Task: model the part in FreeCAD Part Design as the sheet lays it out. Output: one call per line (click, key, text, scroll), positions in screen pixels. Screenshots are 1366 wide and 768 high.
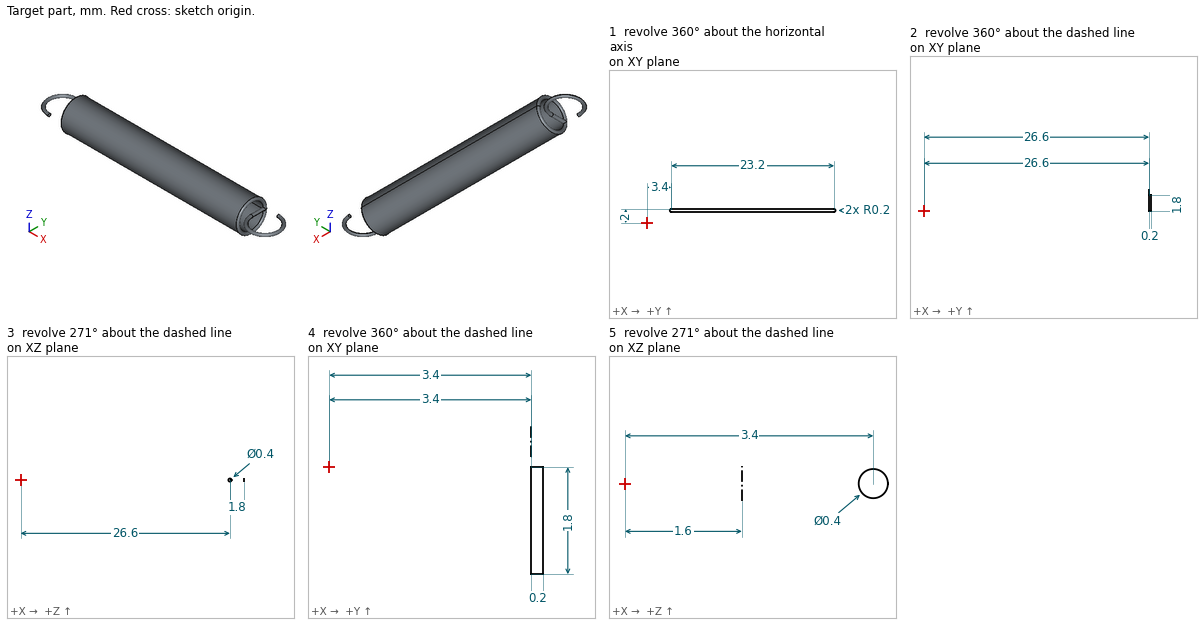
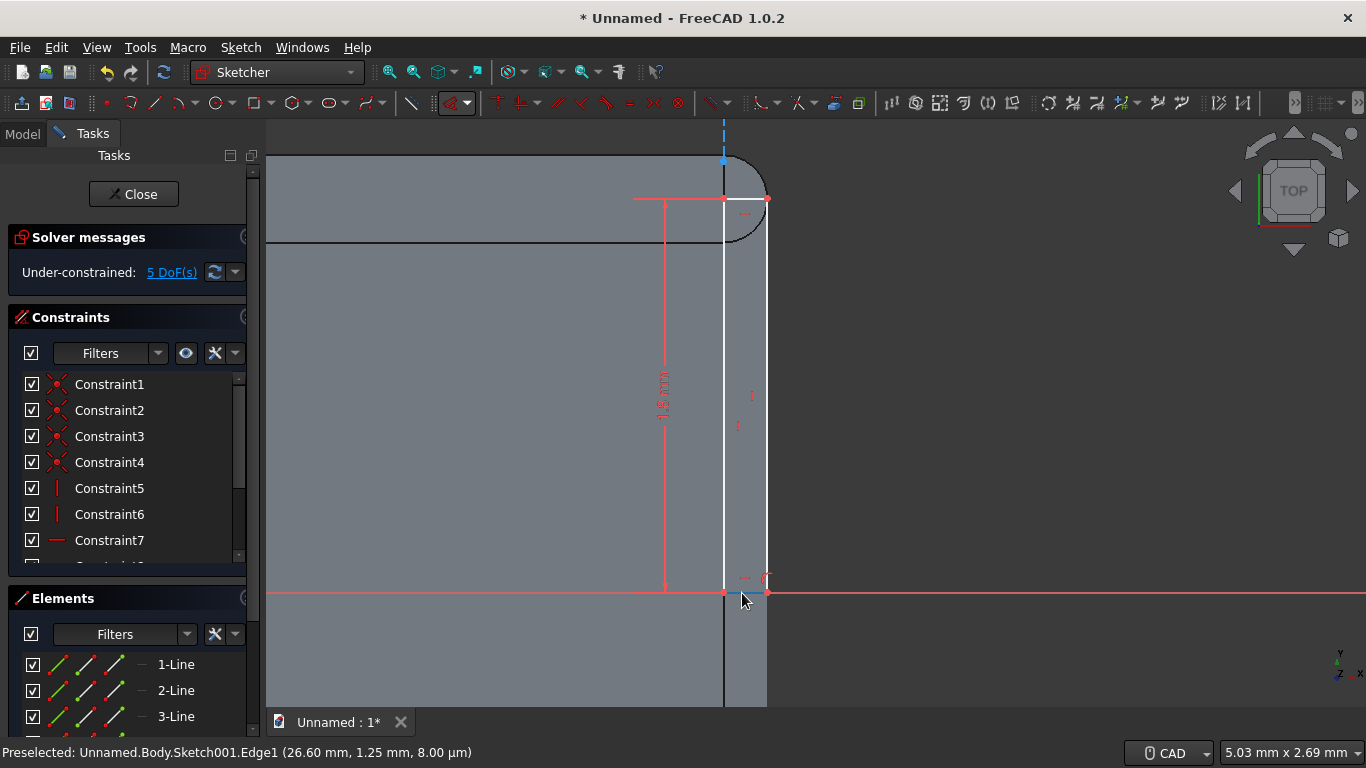
click(741, 593)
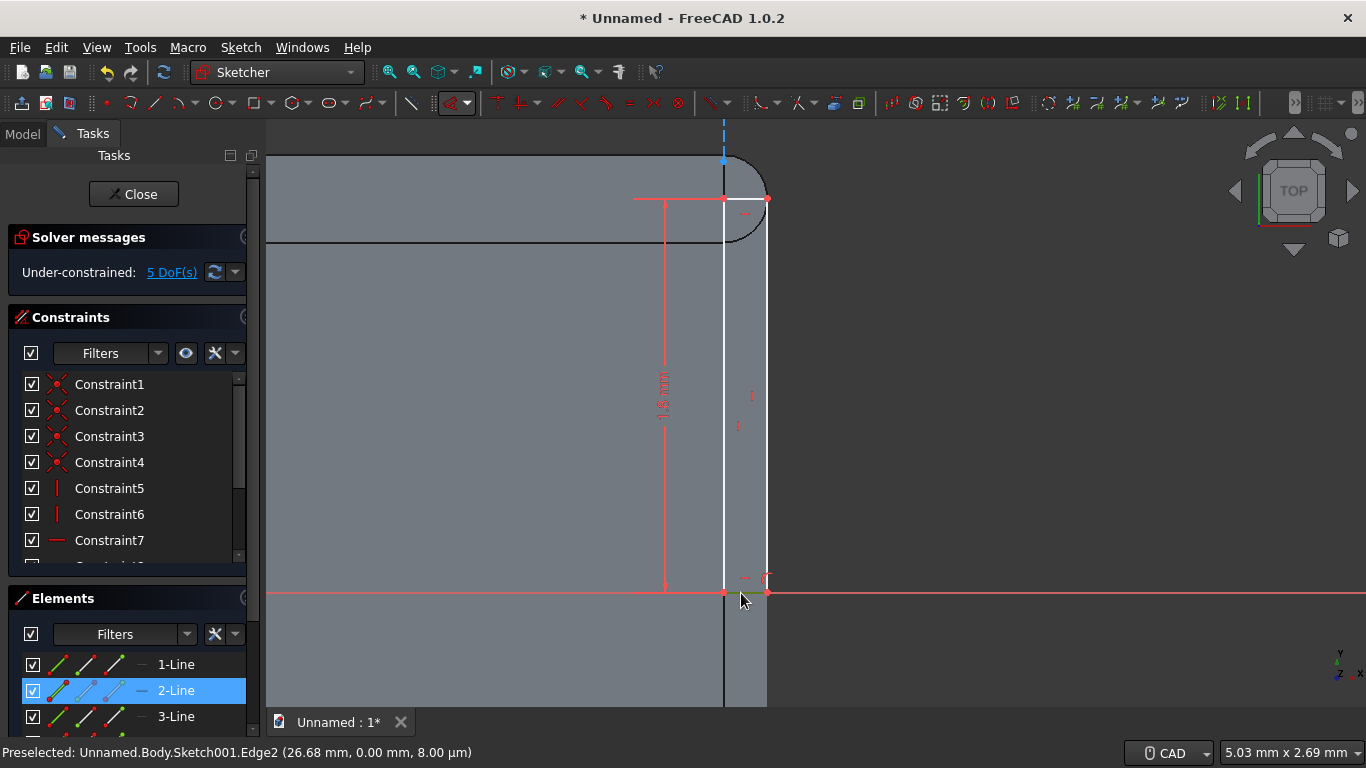
click(470, 104)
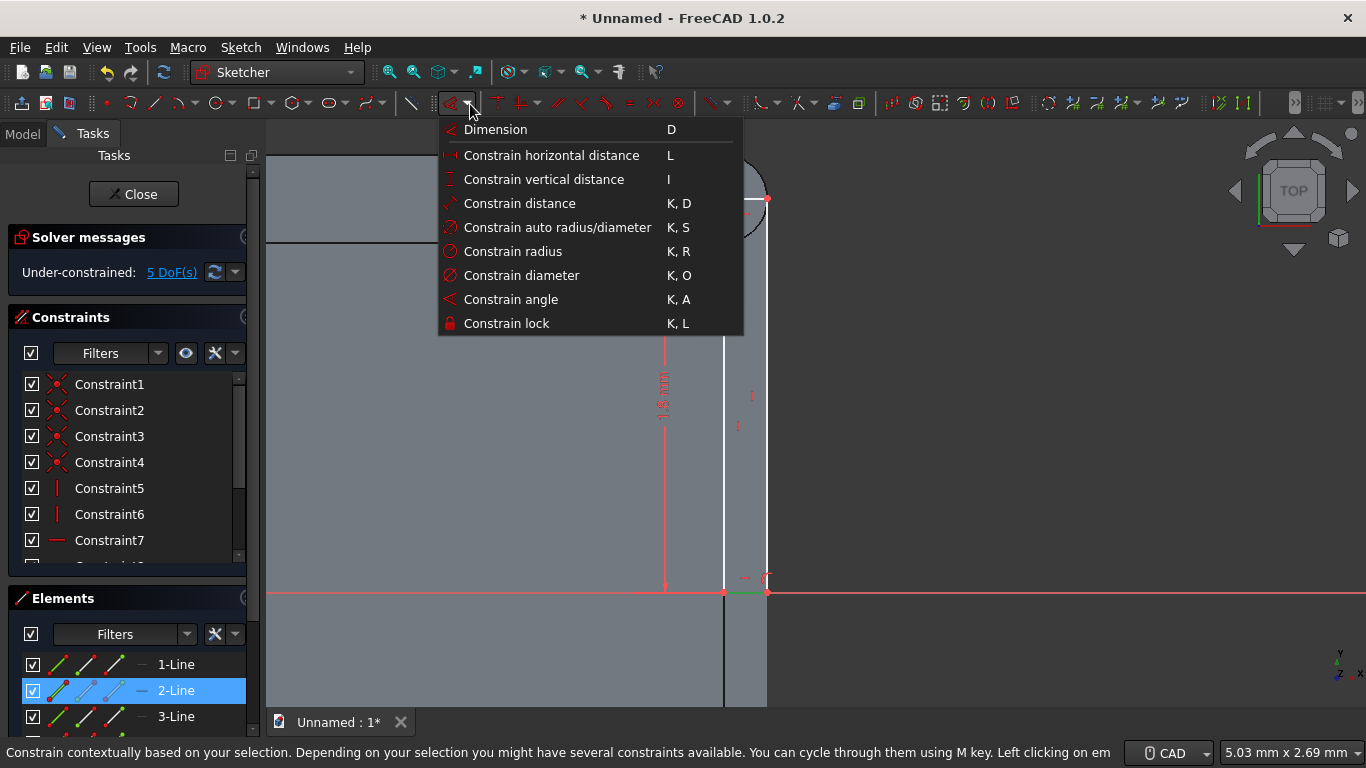
click(591, 155)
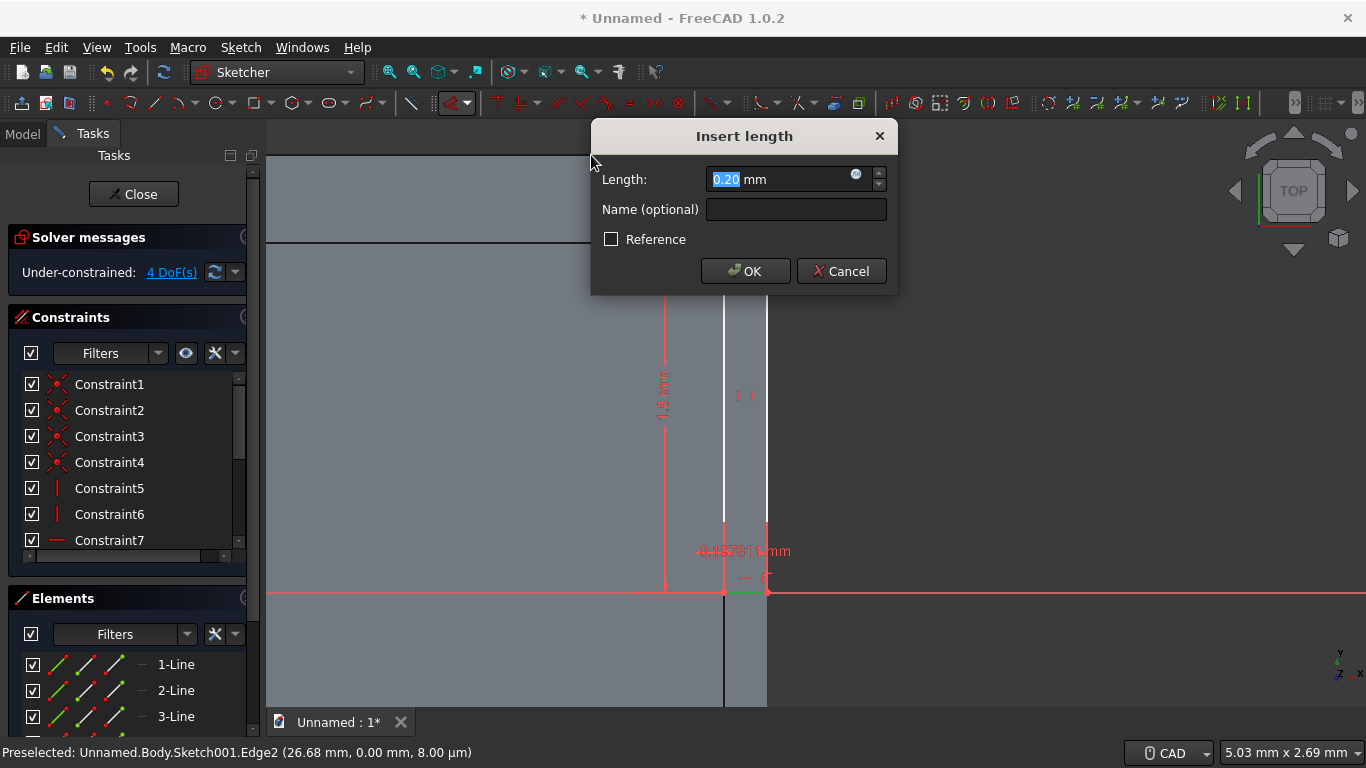
text(0.2)
key(Return)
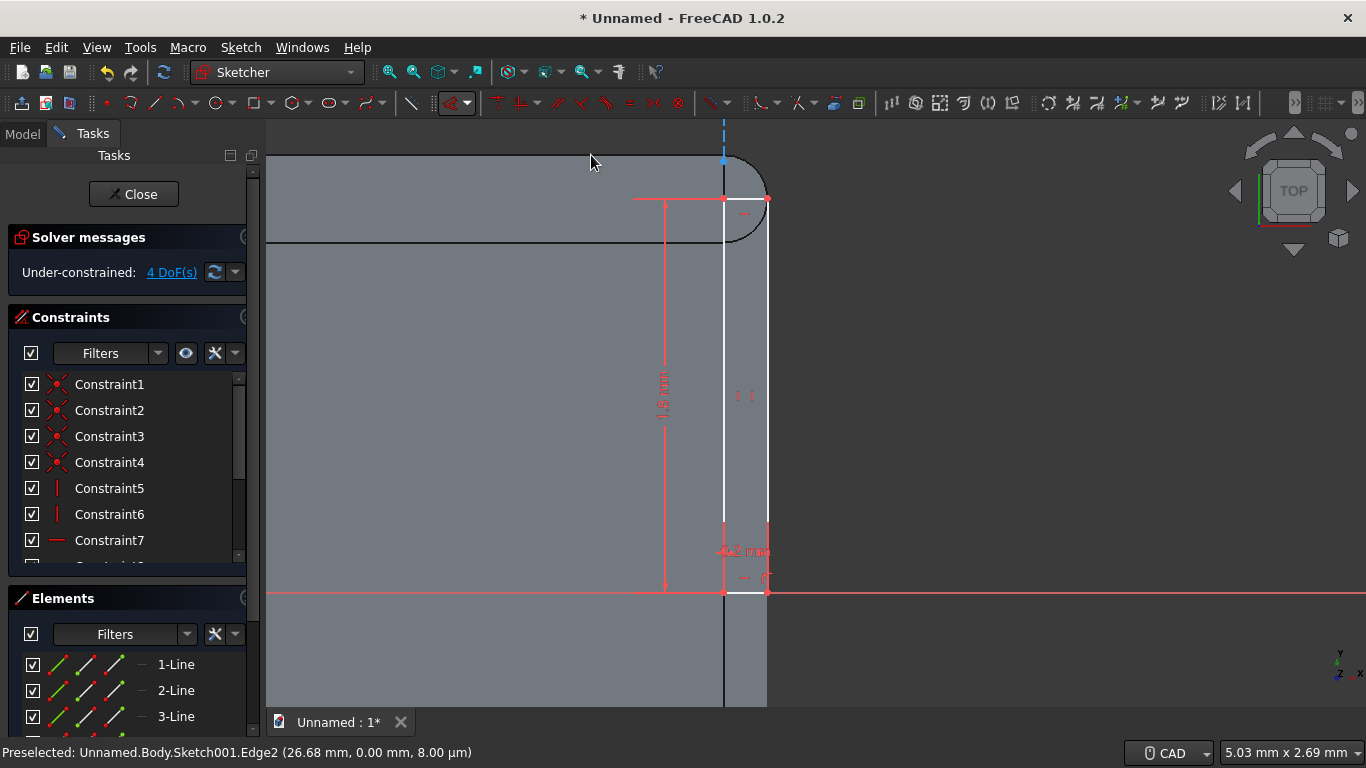
click(724, 199)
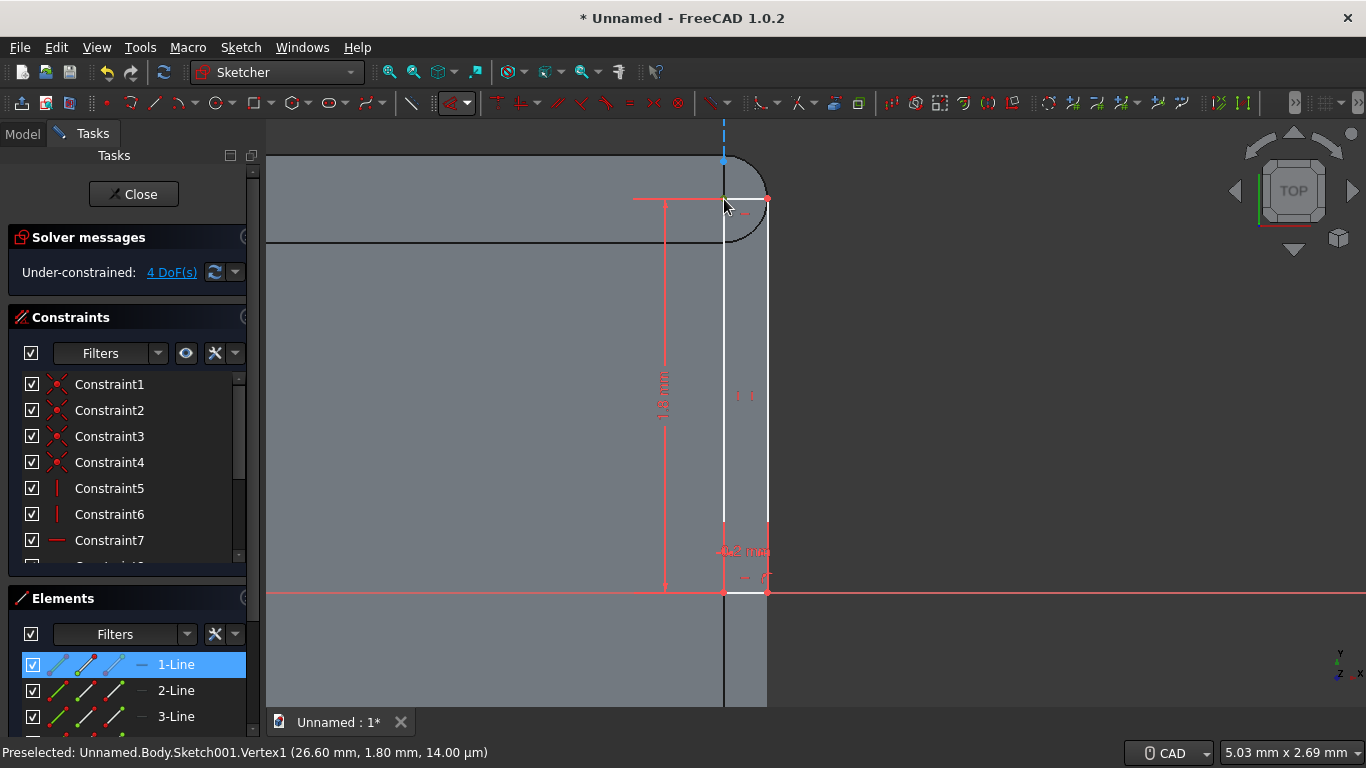
key(l)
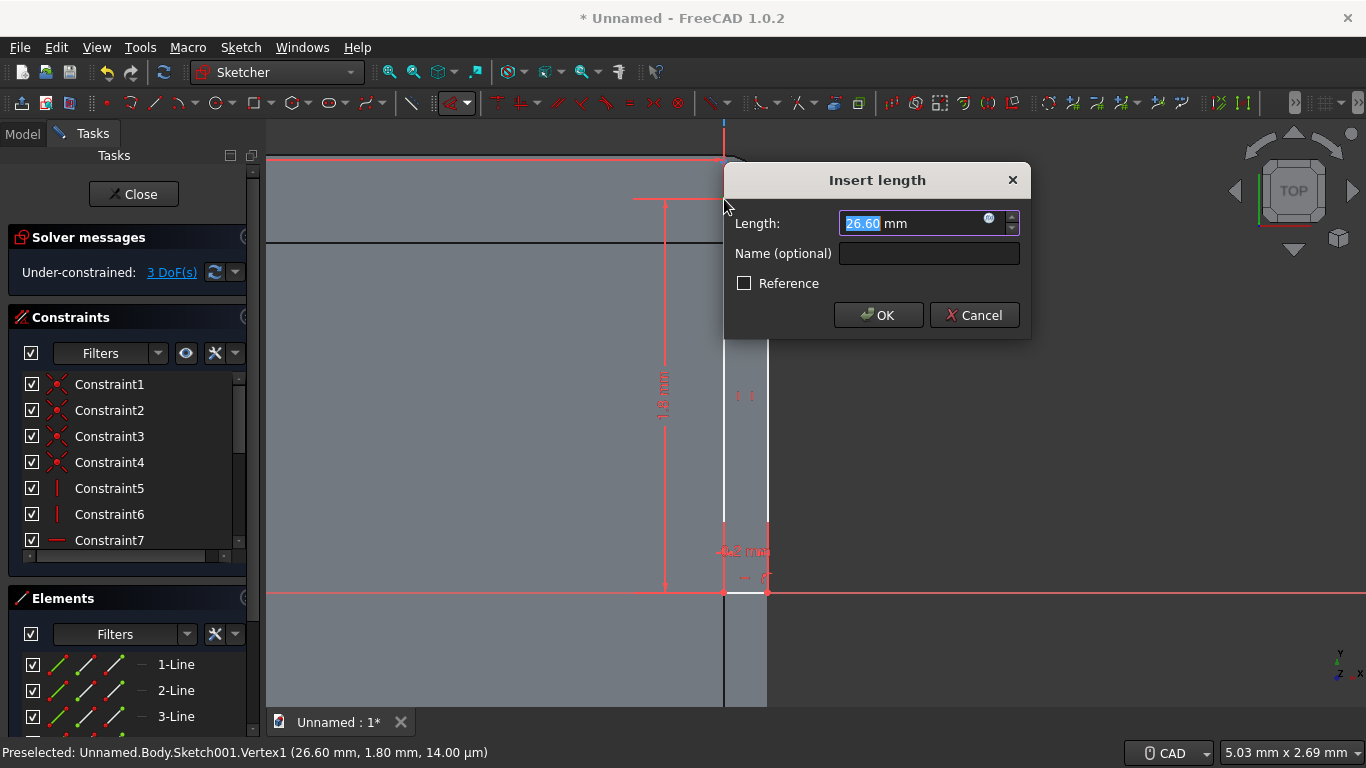
text(26.6)
key(Return)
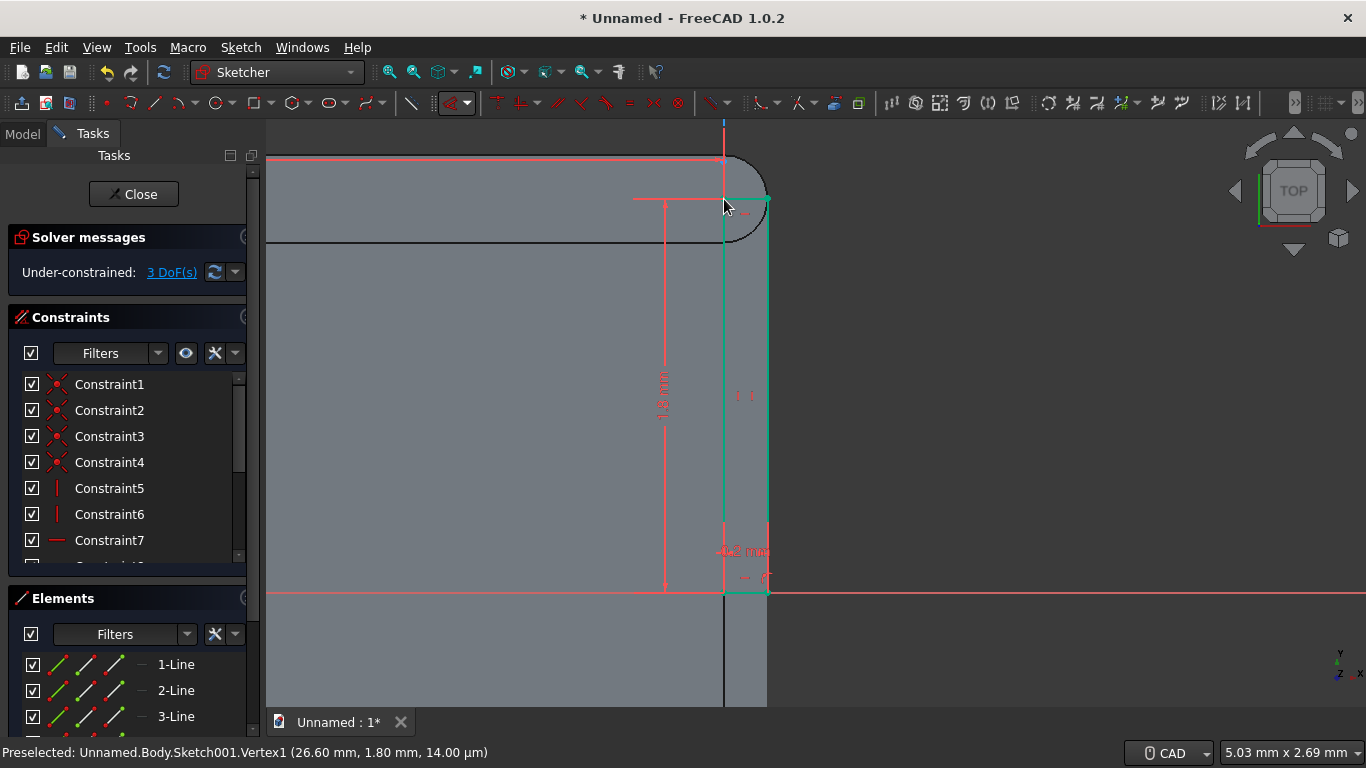
click(724, 161)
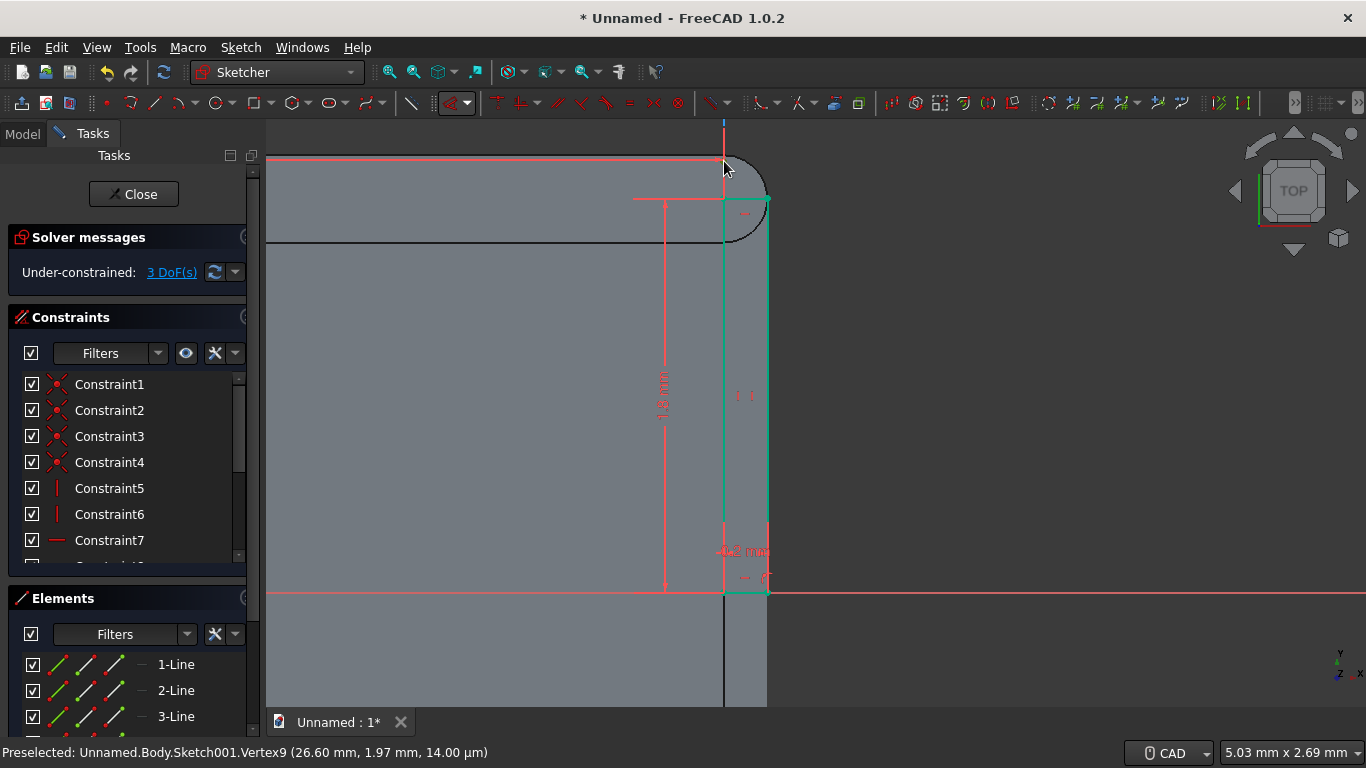
click(470, 104)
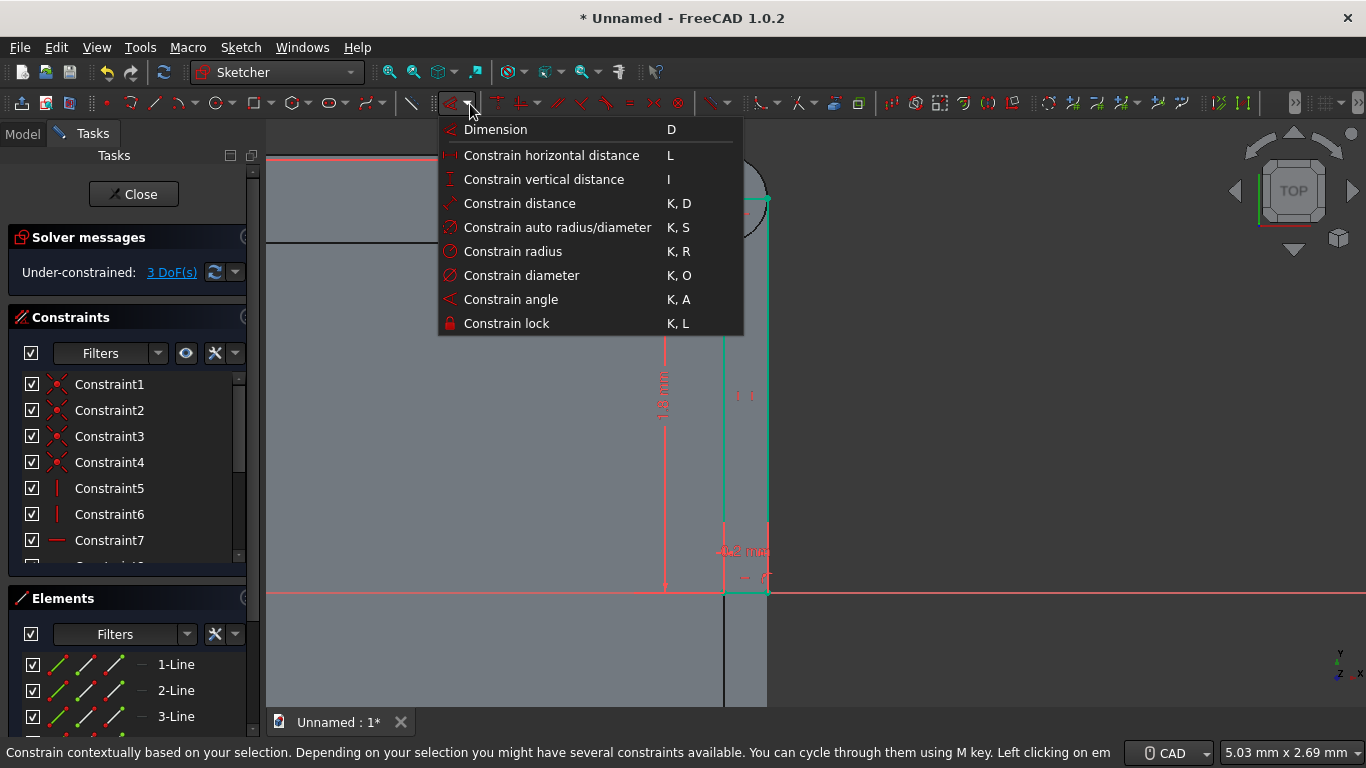
click(591, 155)